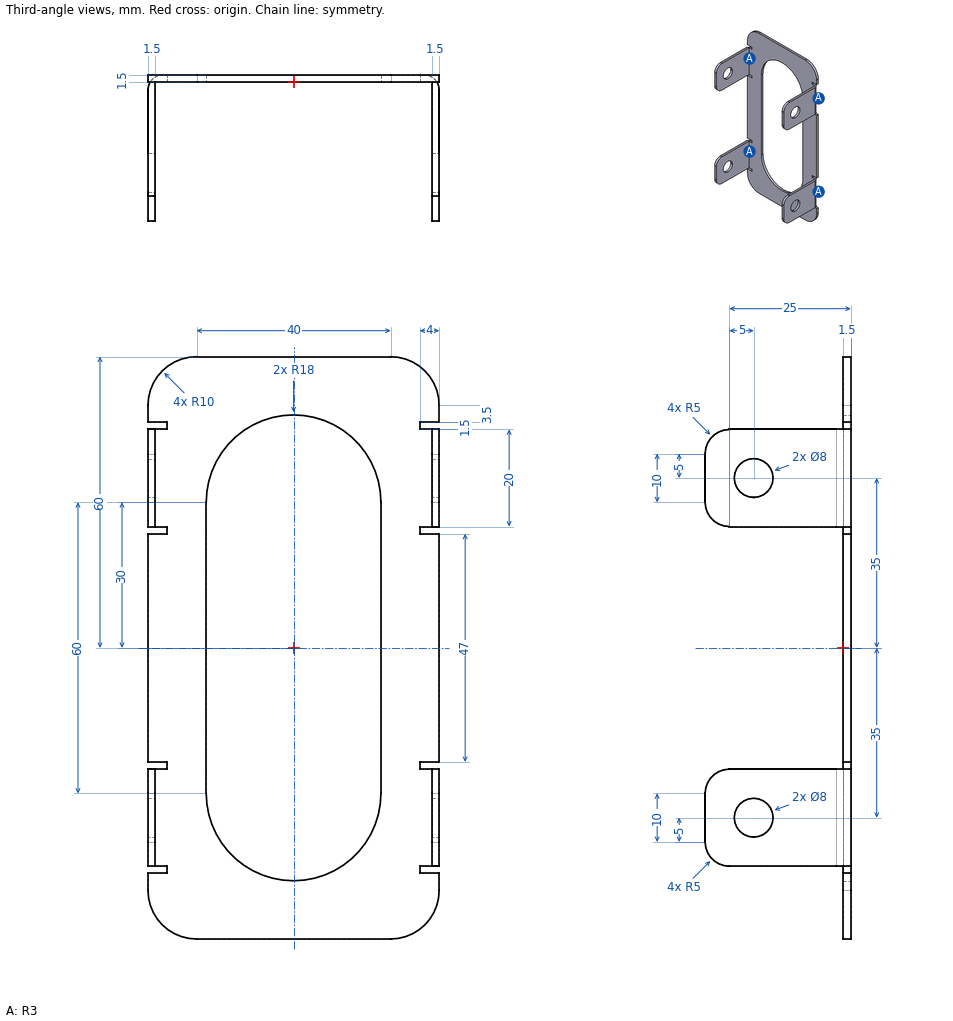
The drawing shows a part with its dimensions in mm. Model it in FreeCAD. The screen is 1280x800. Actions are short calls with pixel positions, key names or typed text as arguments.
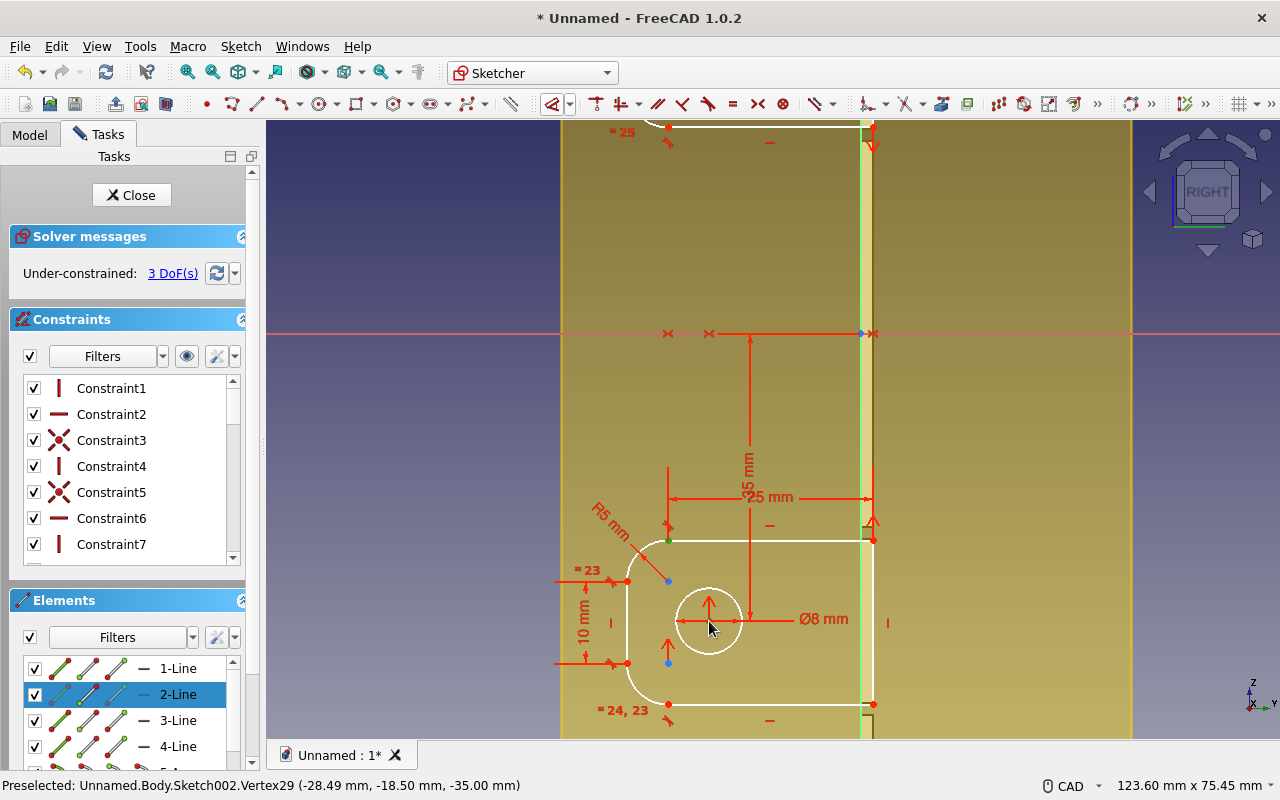
click(570, 104)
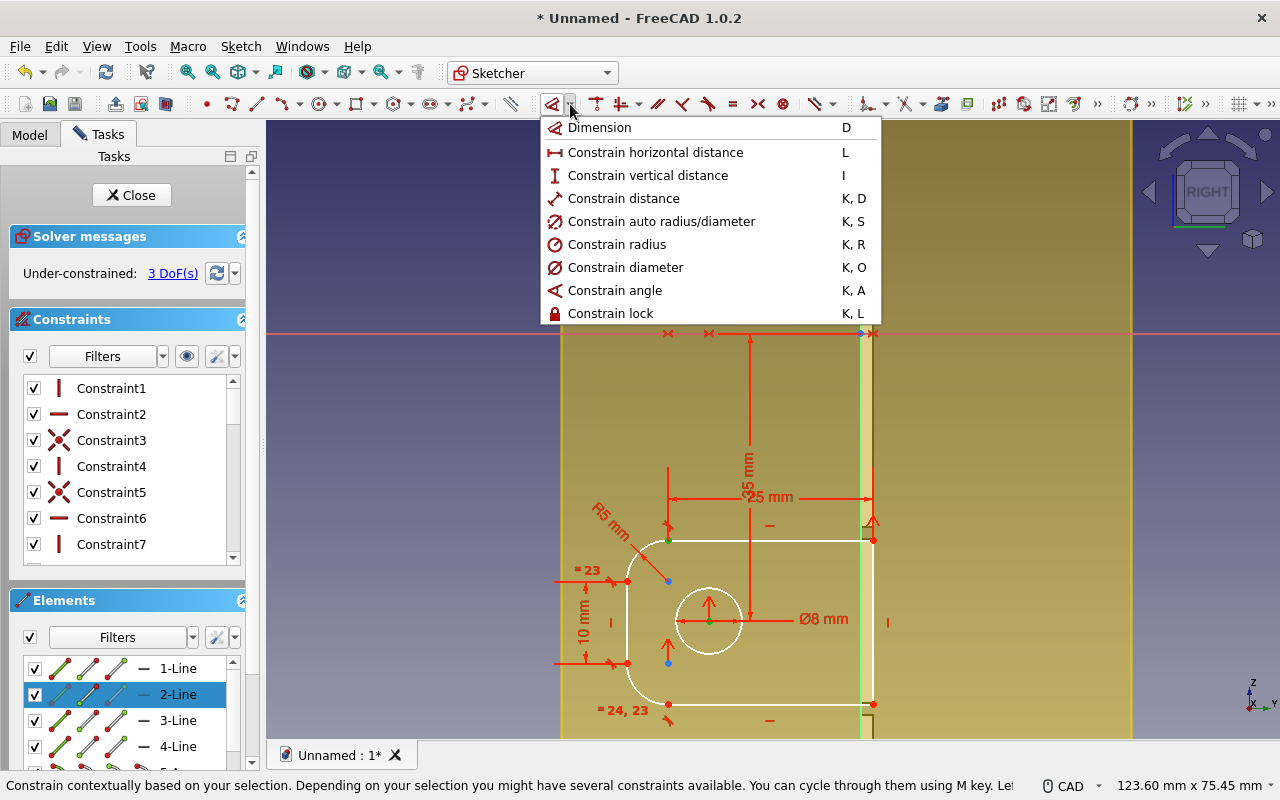
click(711, 152)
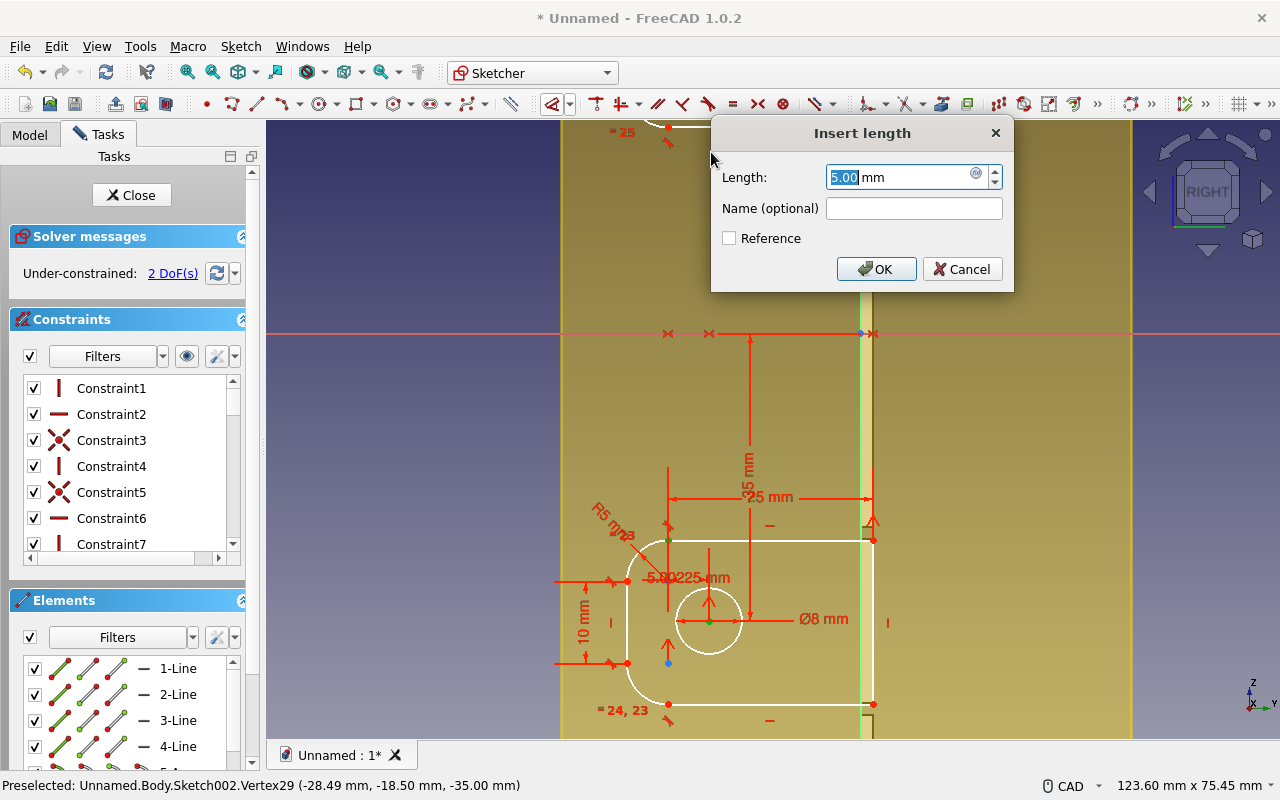
text(5)
key(Return)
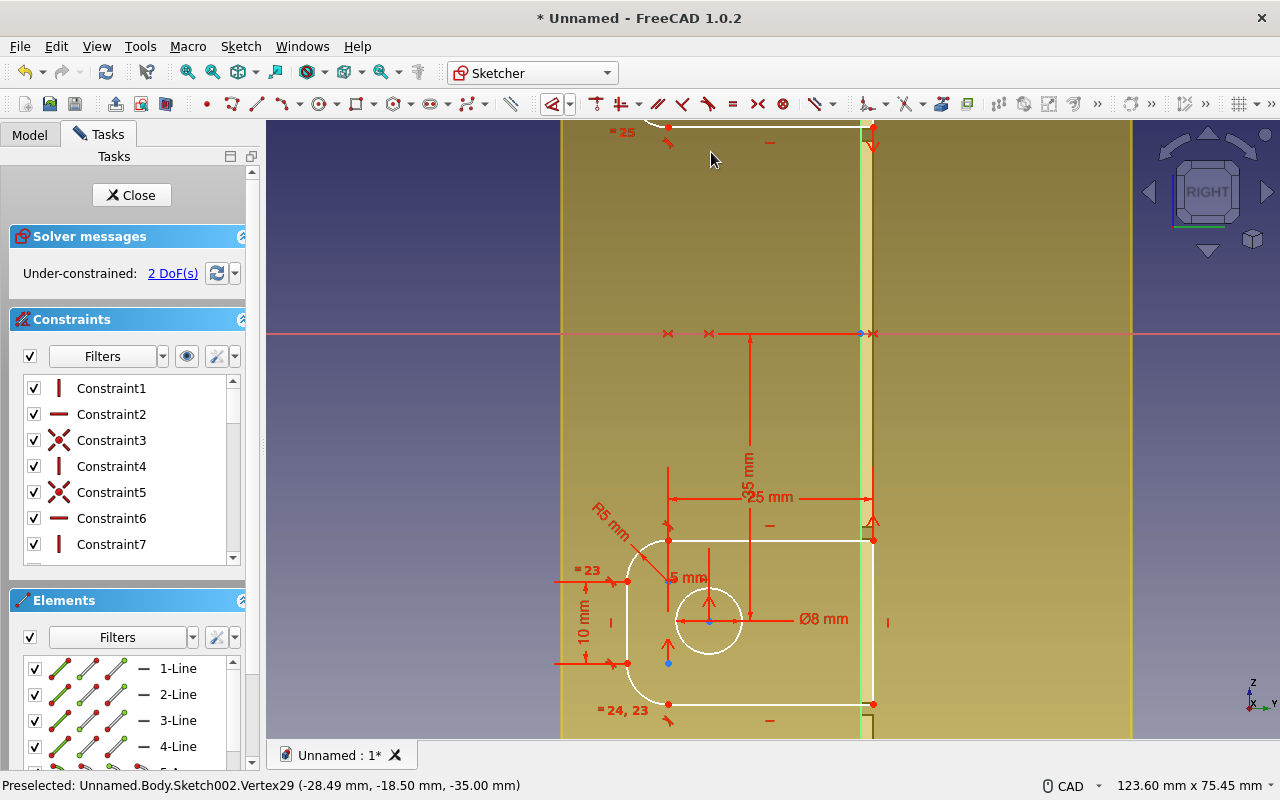
click(627, 664)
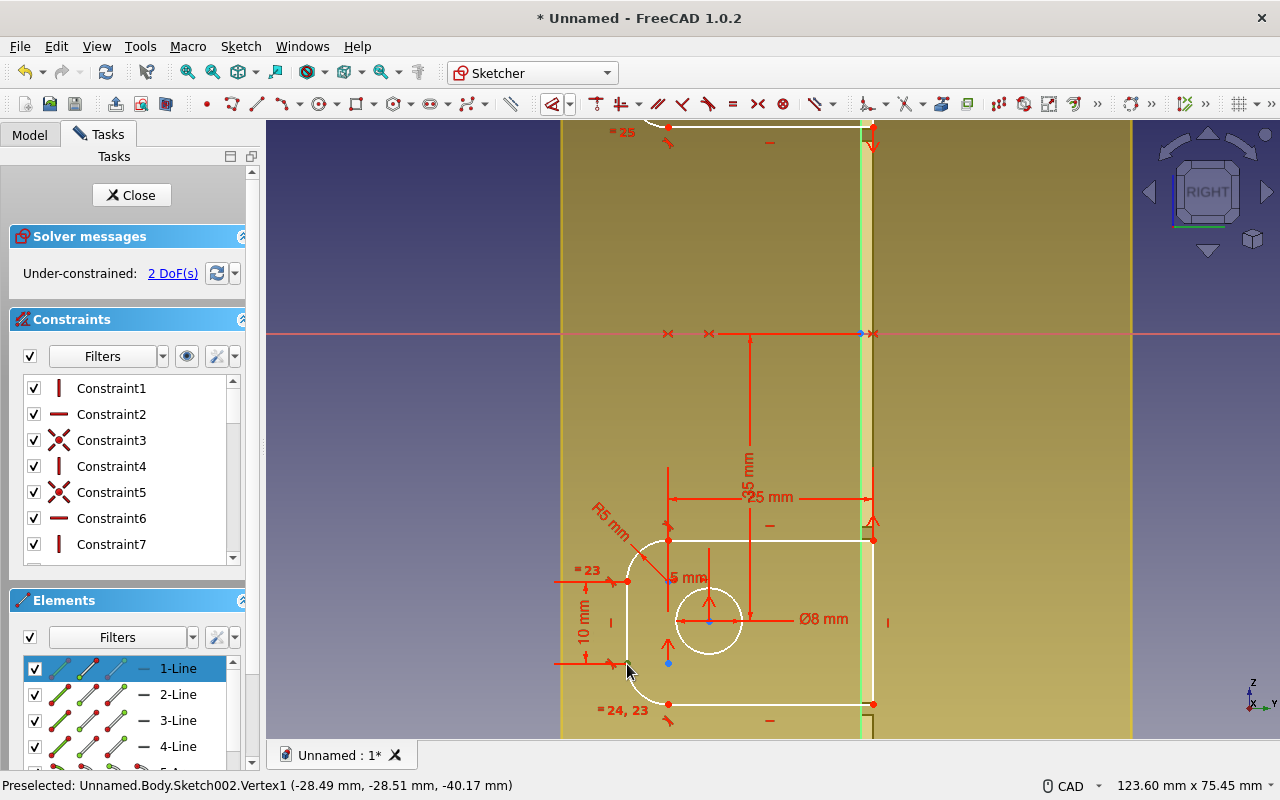
click(709, 621)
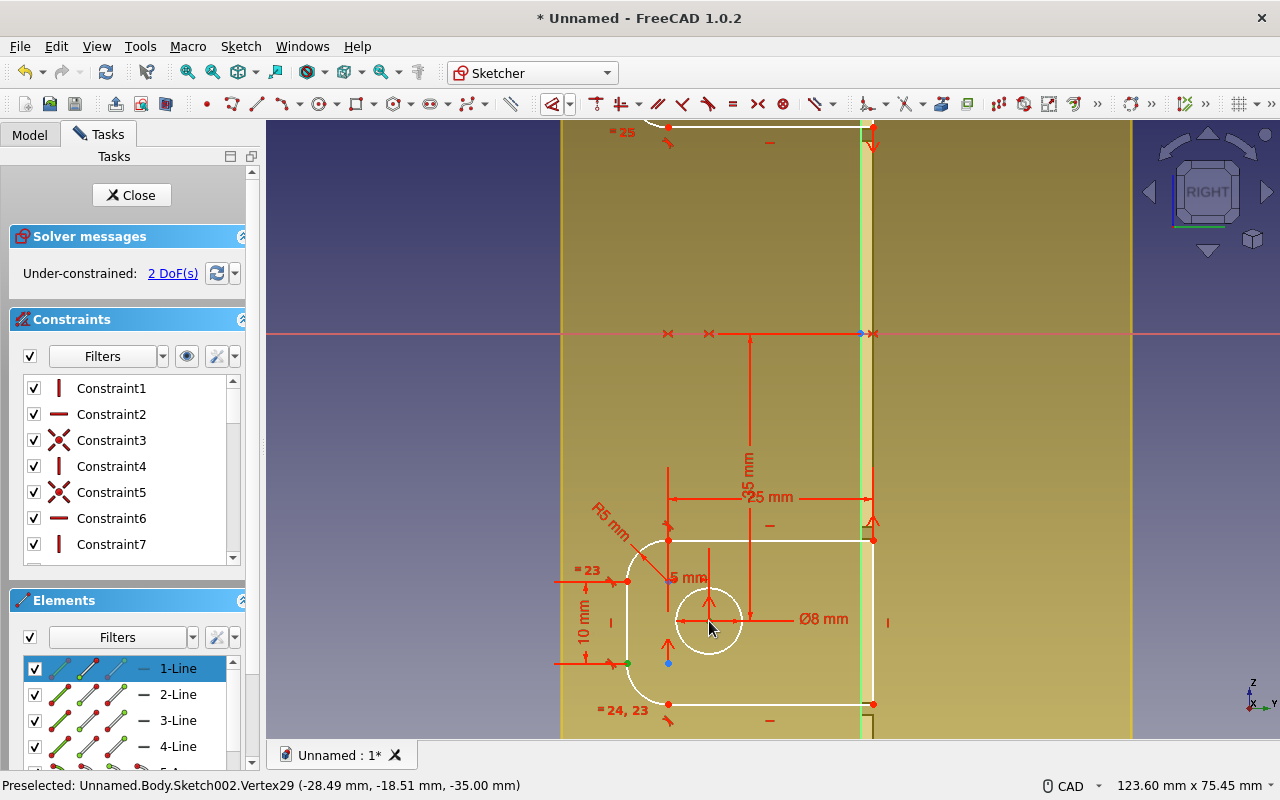
key(i)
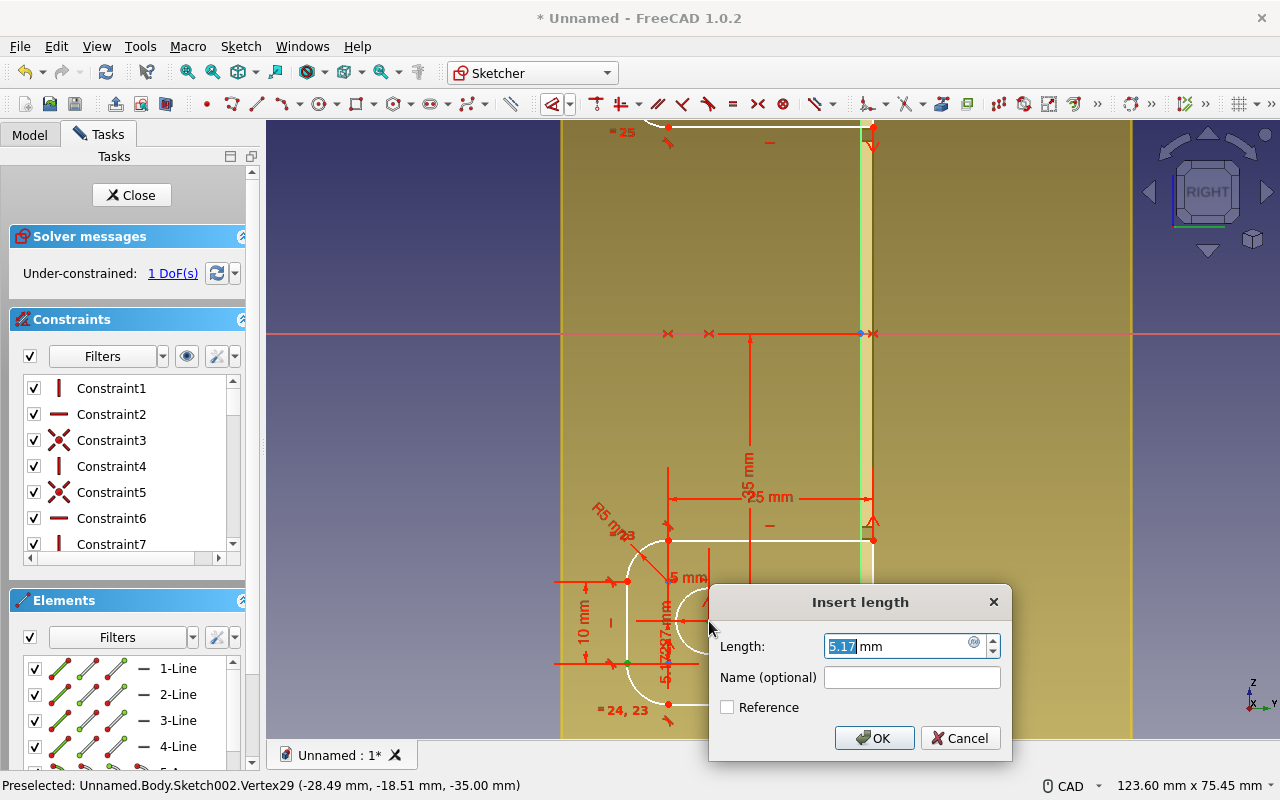
text(5)
key(Return)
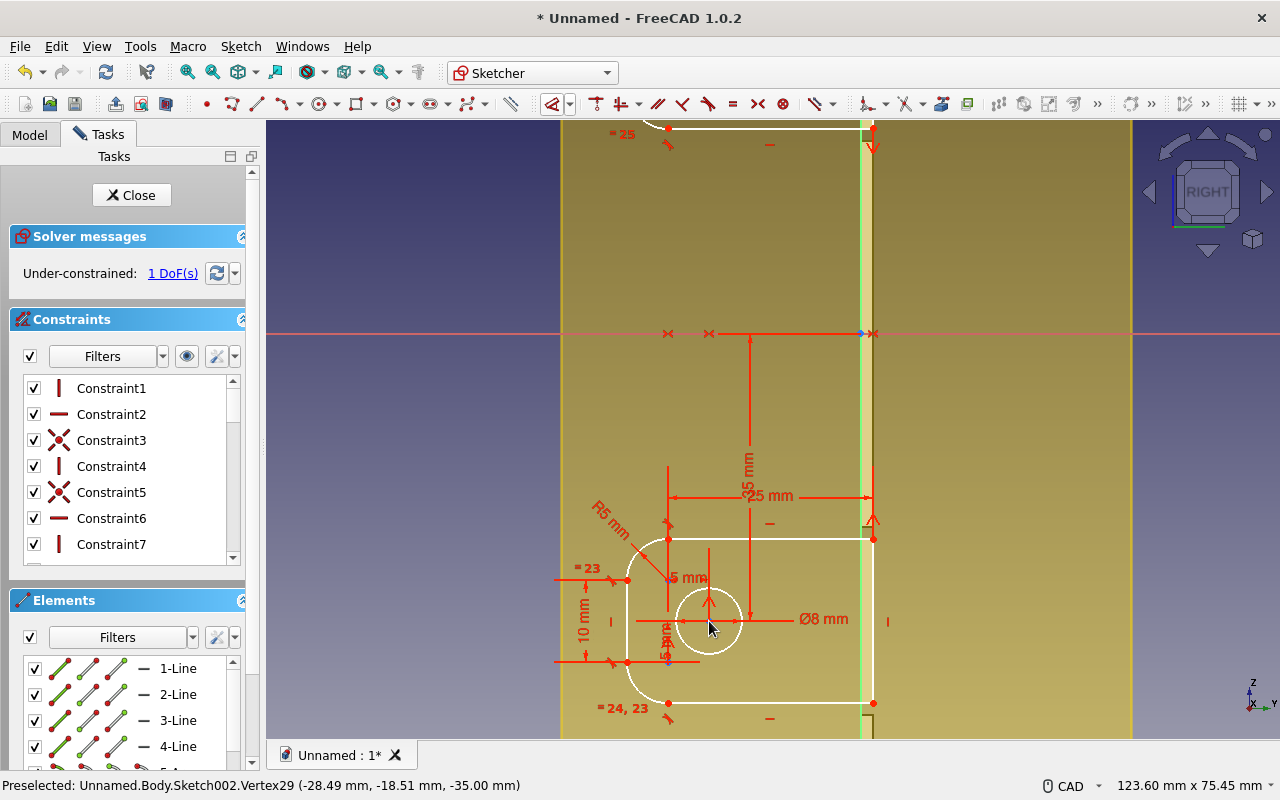
scroll(873, 539, up, 6)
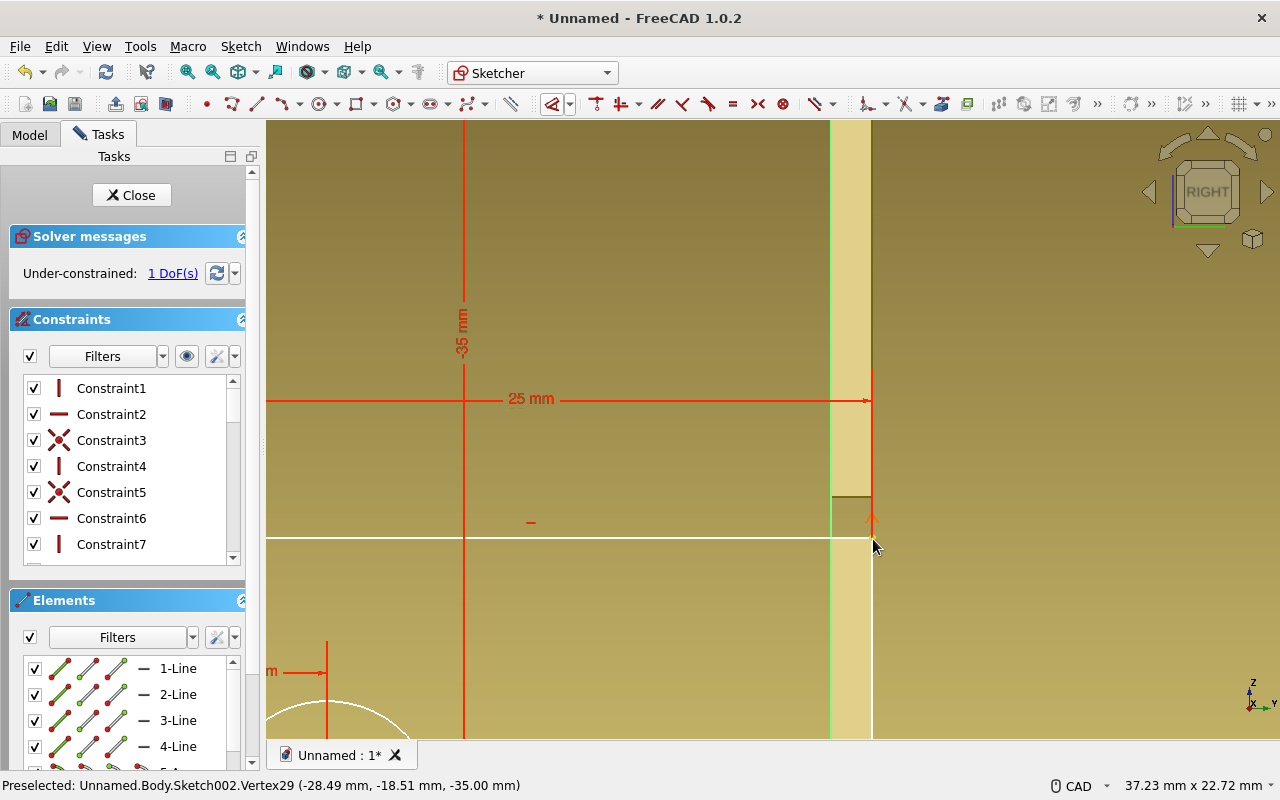
click(872, 538)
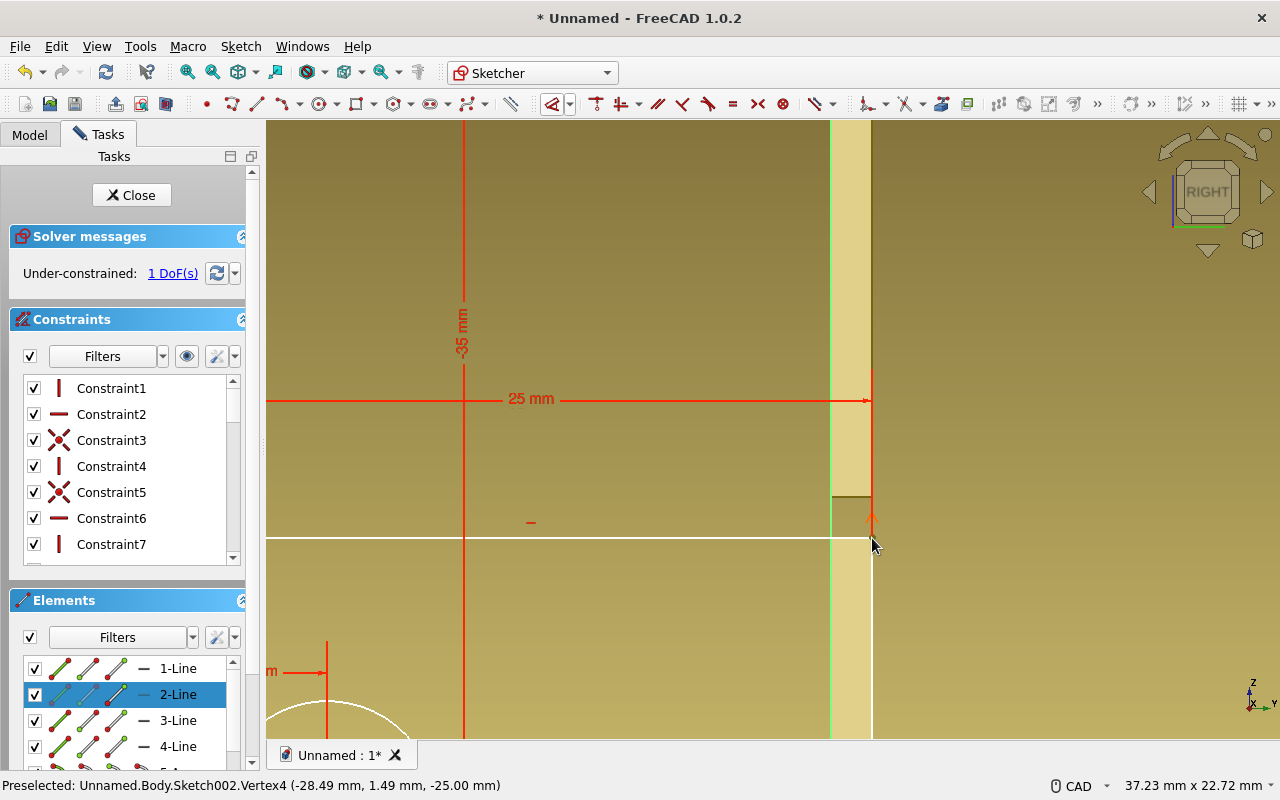
key(l)